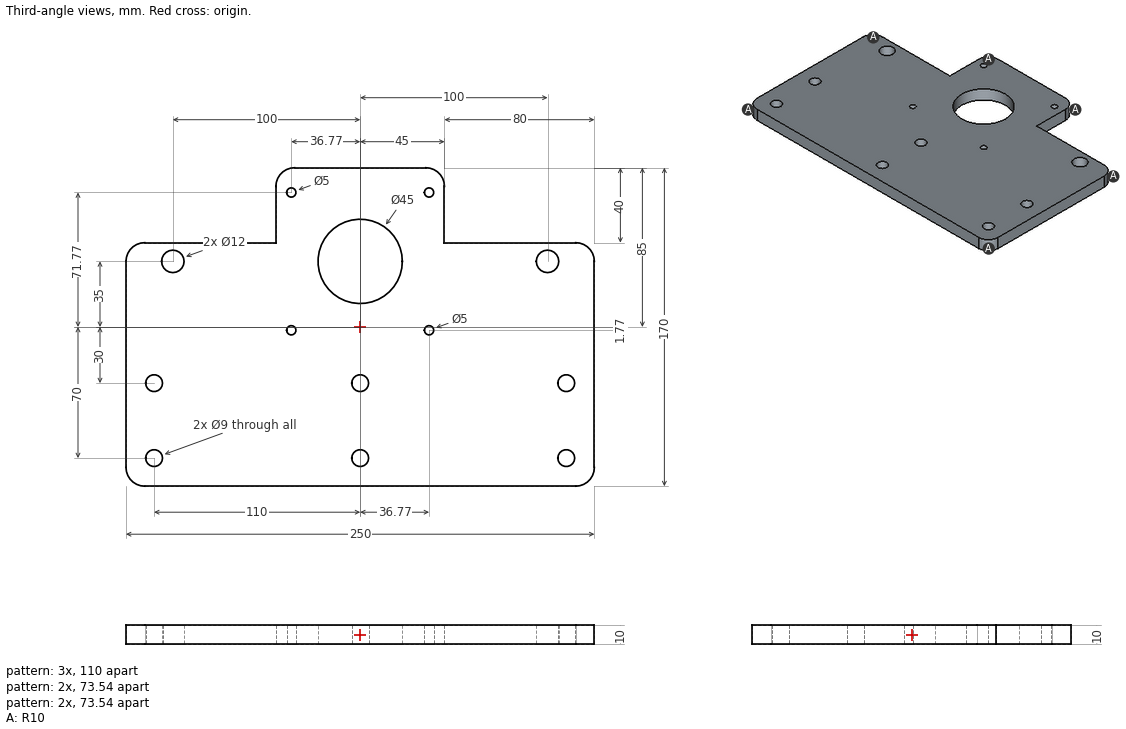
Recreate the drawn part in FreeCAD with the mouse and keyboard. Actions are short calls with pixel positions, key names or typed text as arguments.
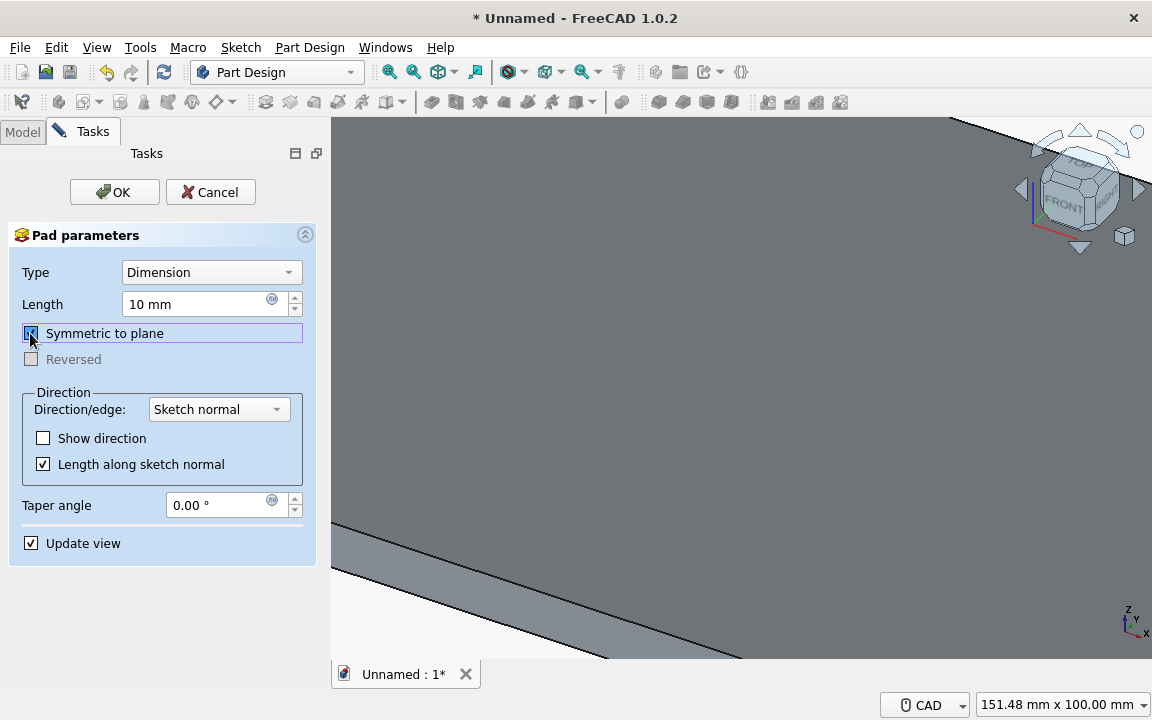
click(115, 192)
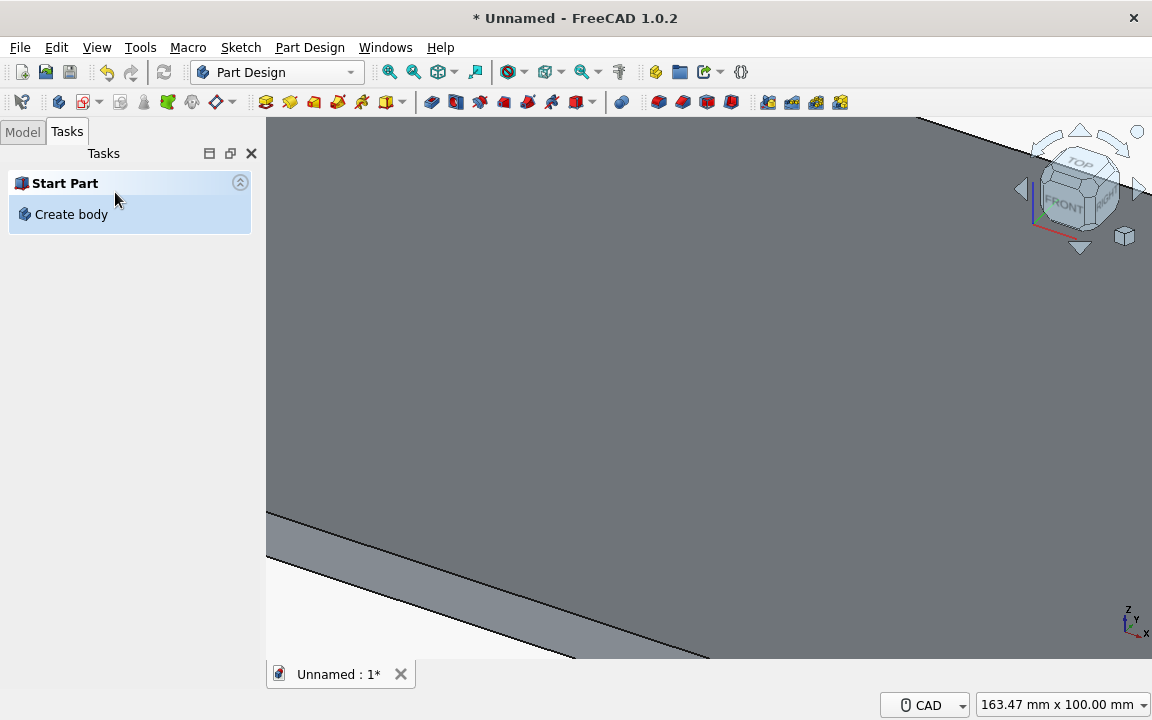
key(v)
key(f)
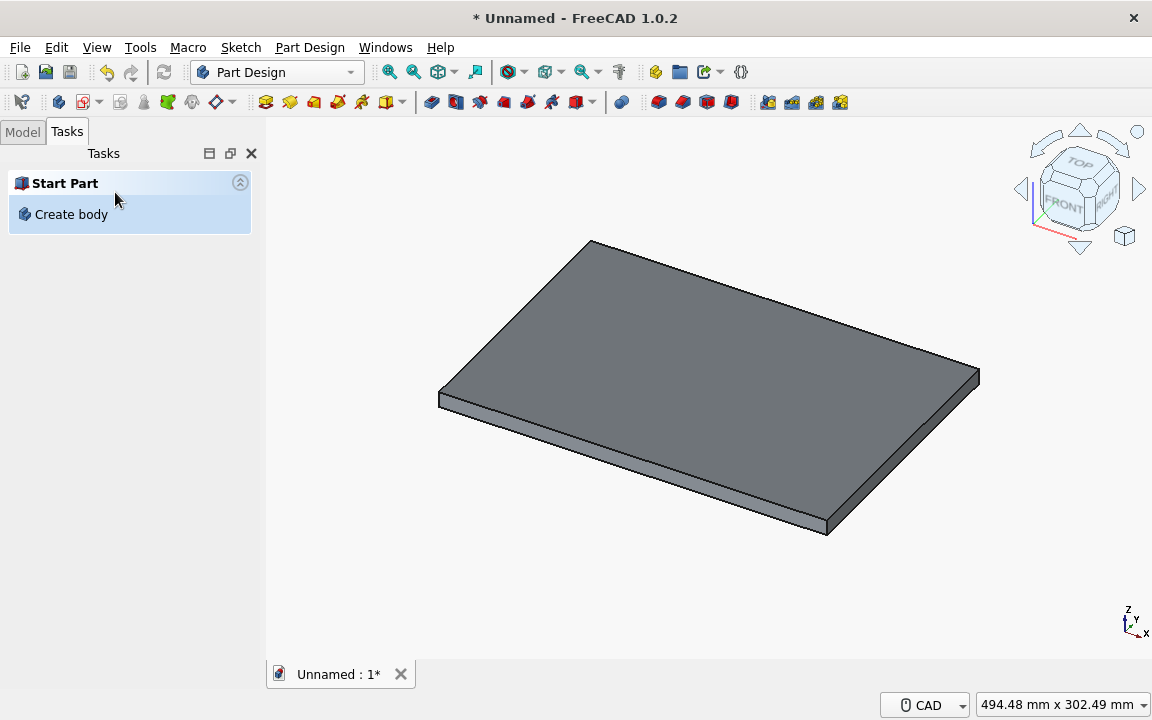
click(764, 398)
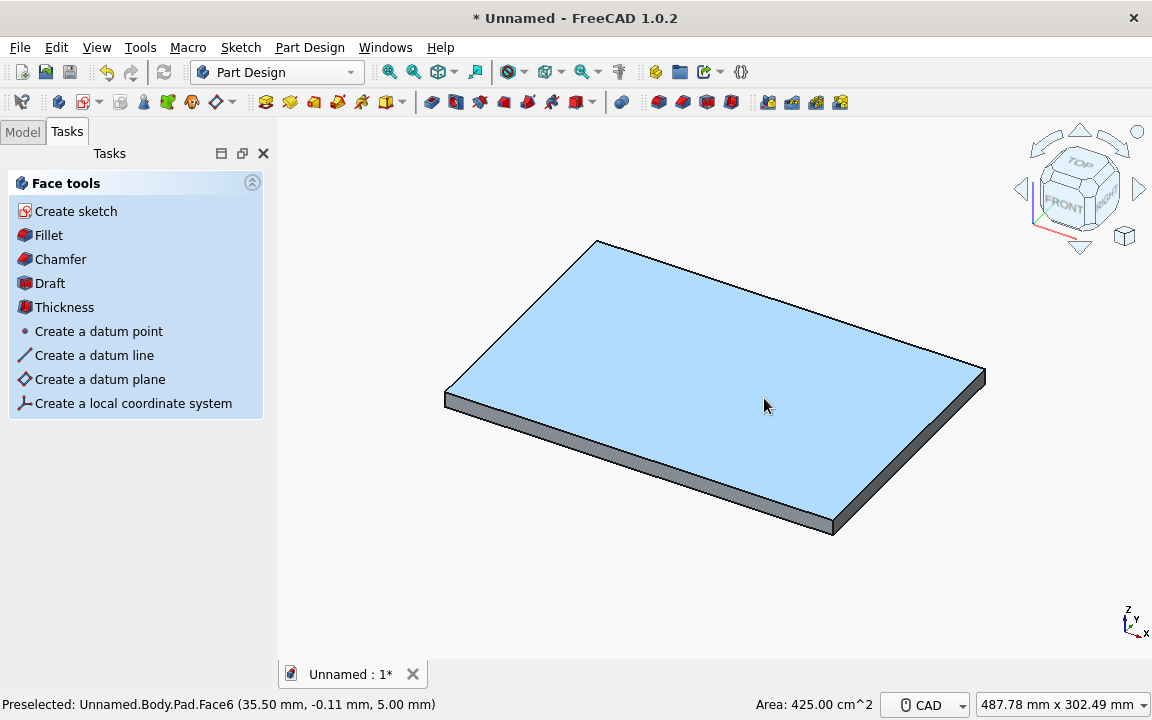
click(84, 102)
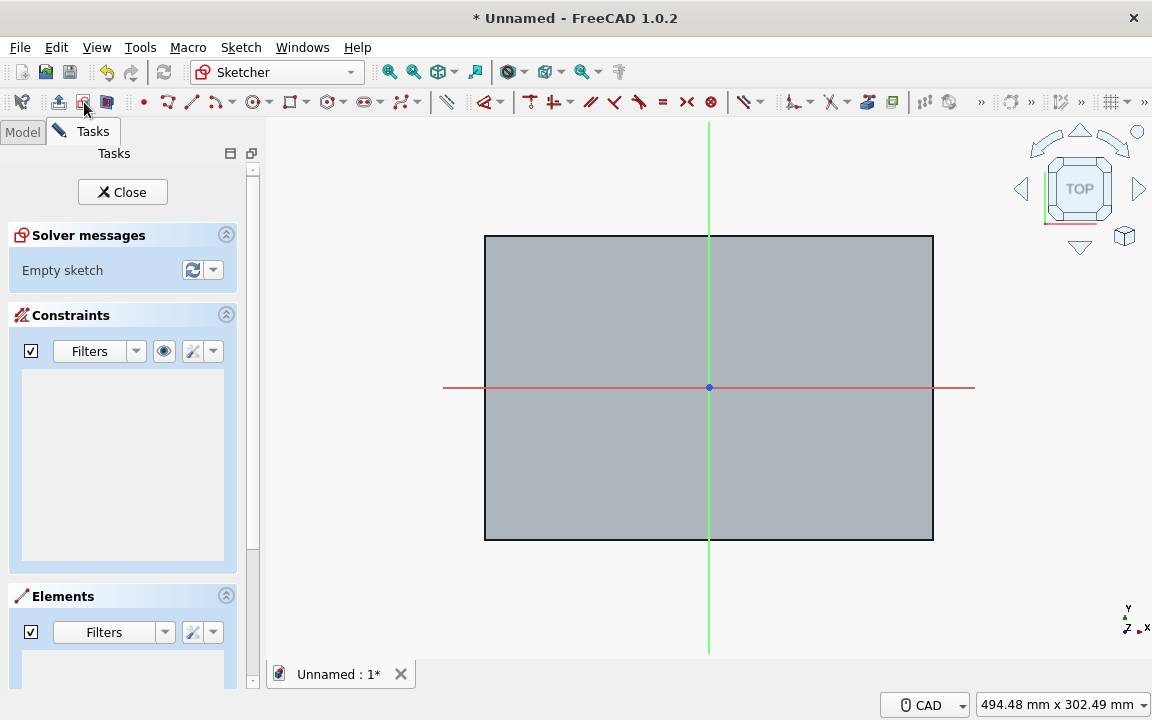
scroll(968, 250, up, 4)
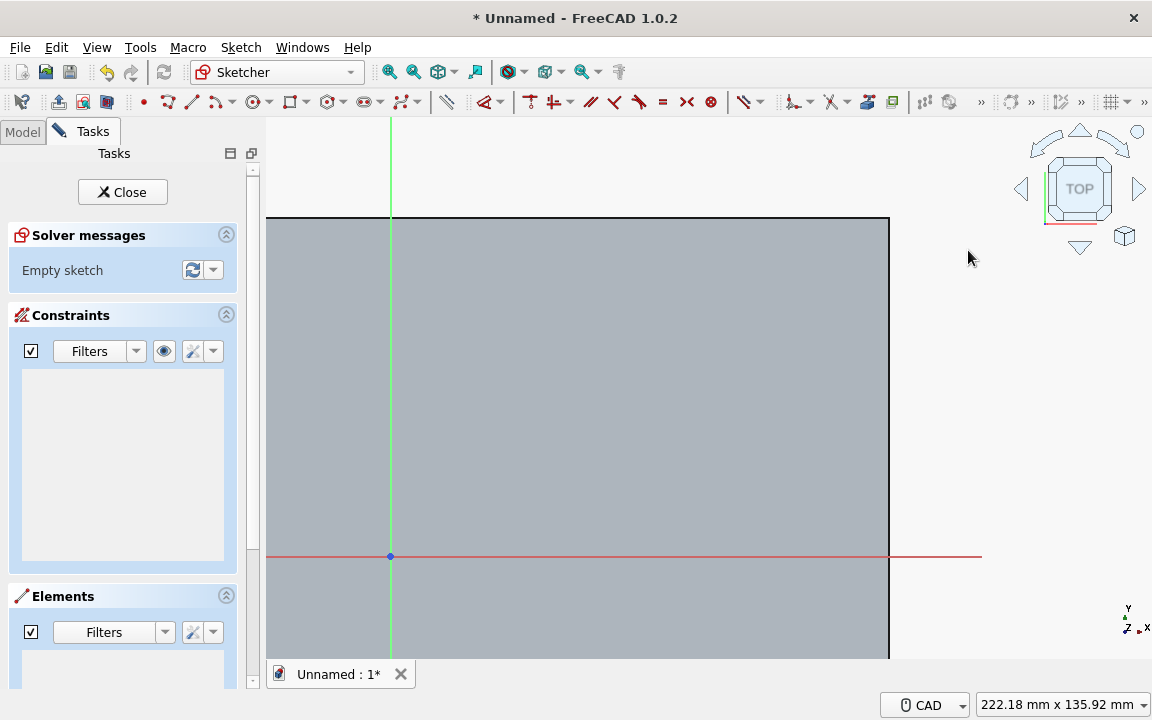
key(g)
key(r)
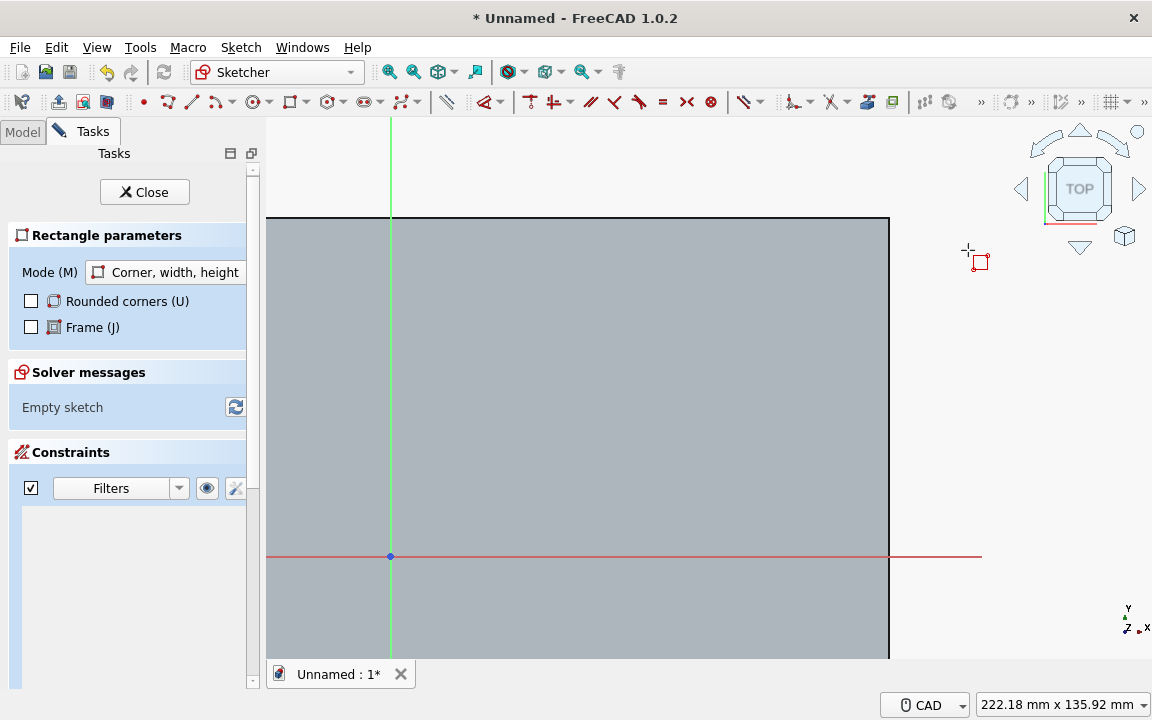
click(570, 218)
move(889, 377)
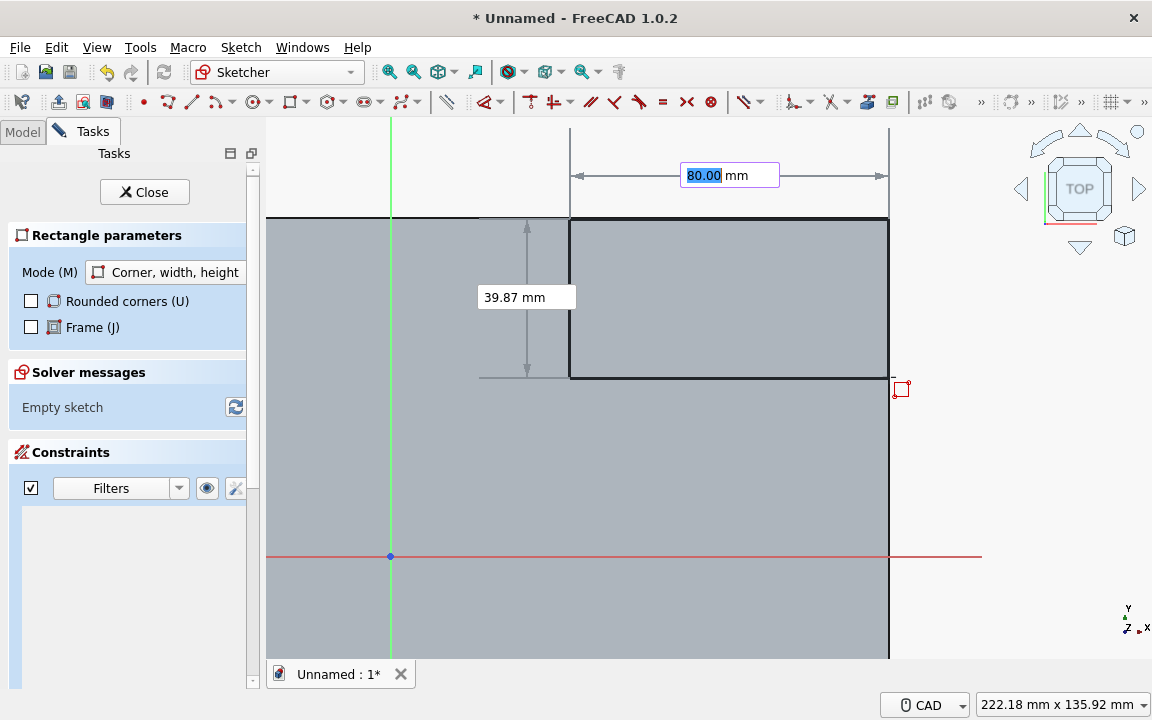
text(80)
key(Tab)
text(40)
key(Return)
key(Escape)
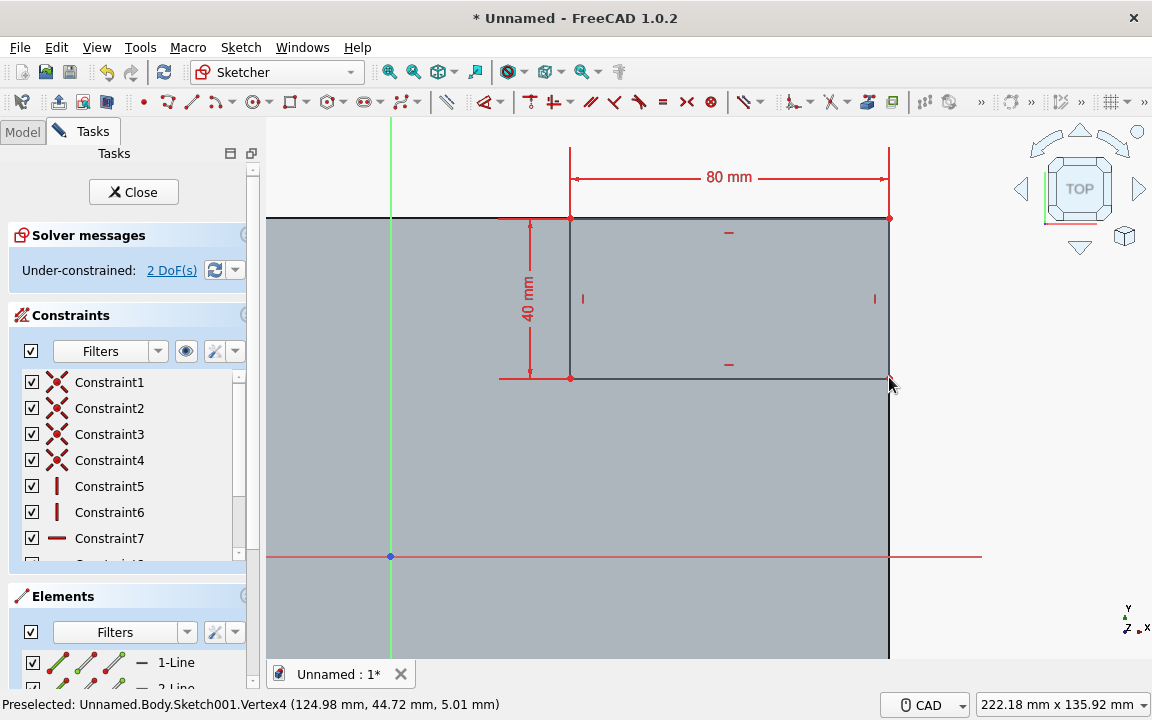
key(d)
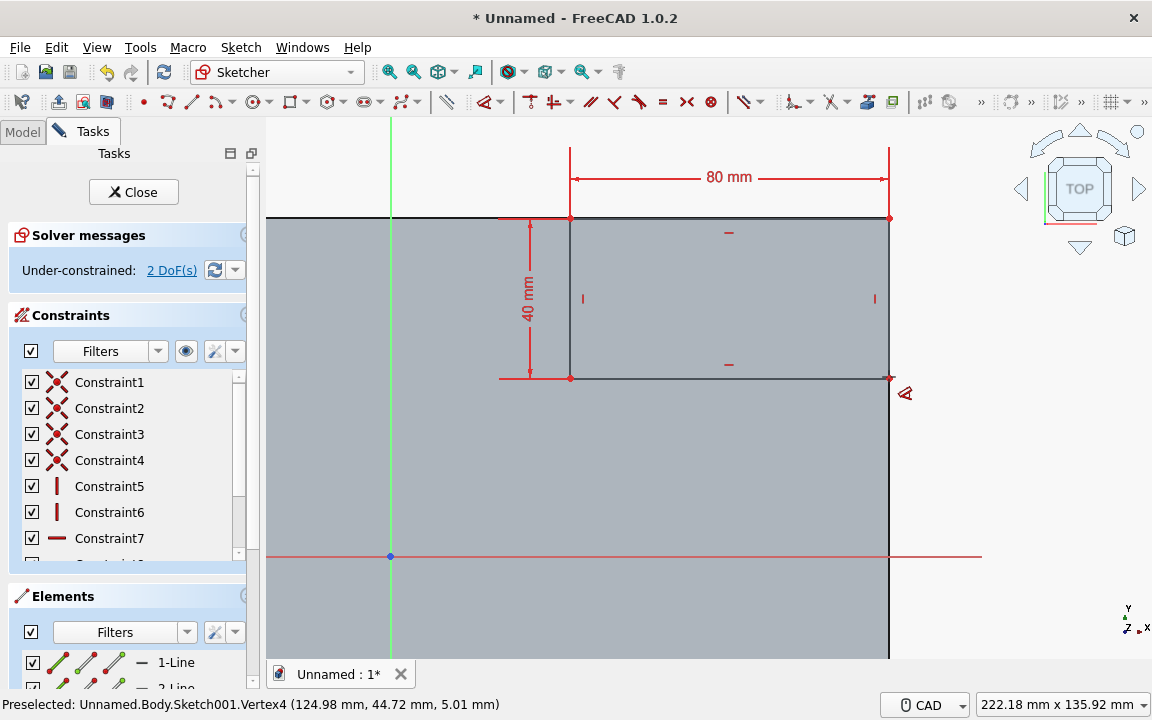
click(570, 219)
click(480, 591)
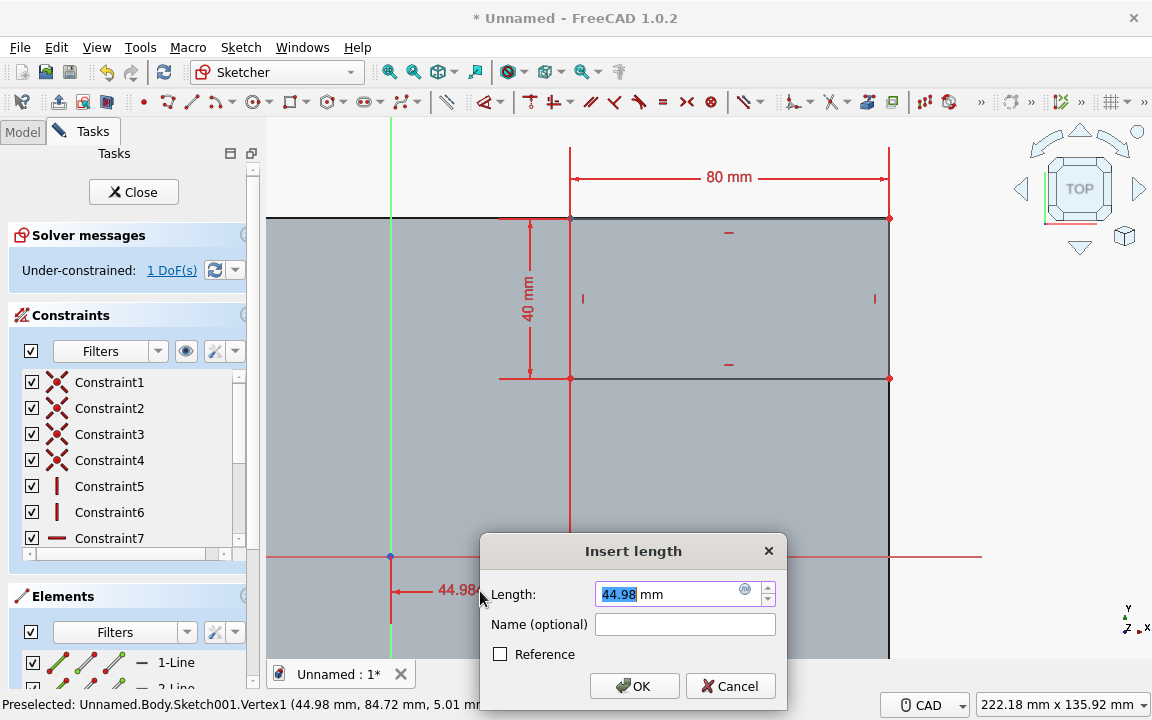
text(45)
key(Return)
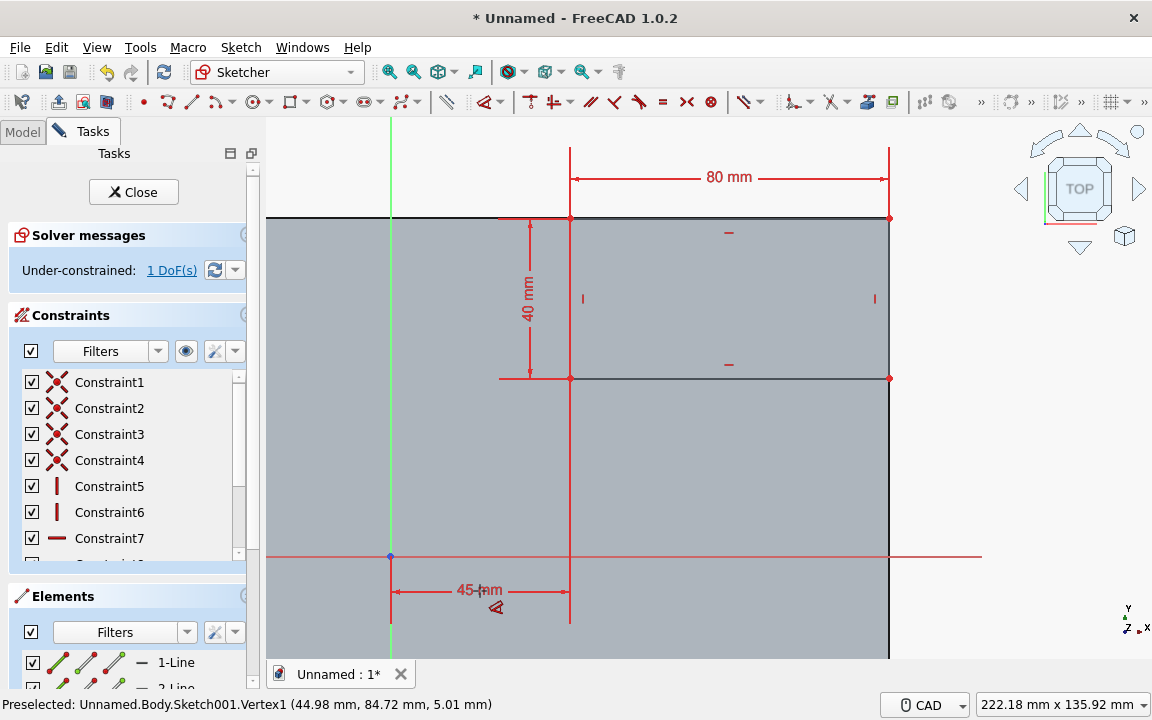
click(570, 219)
click(357, 388)